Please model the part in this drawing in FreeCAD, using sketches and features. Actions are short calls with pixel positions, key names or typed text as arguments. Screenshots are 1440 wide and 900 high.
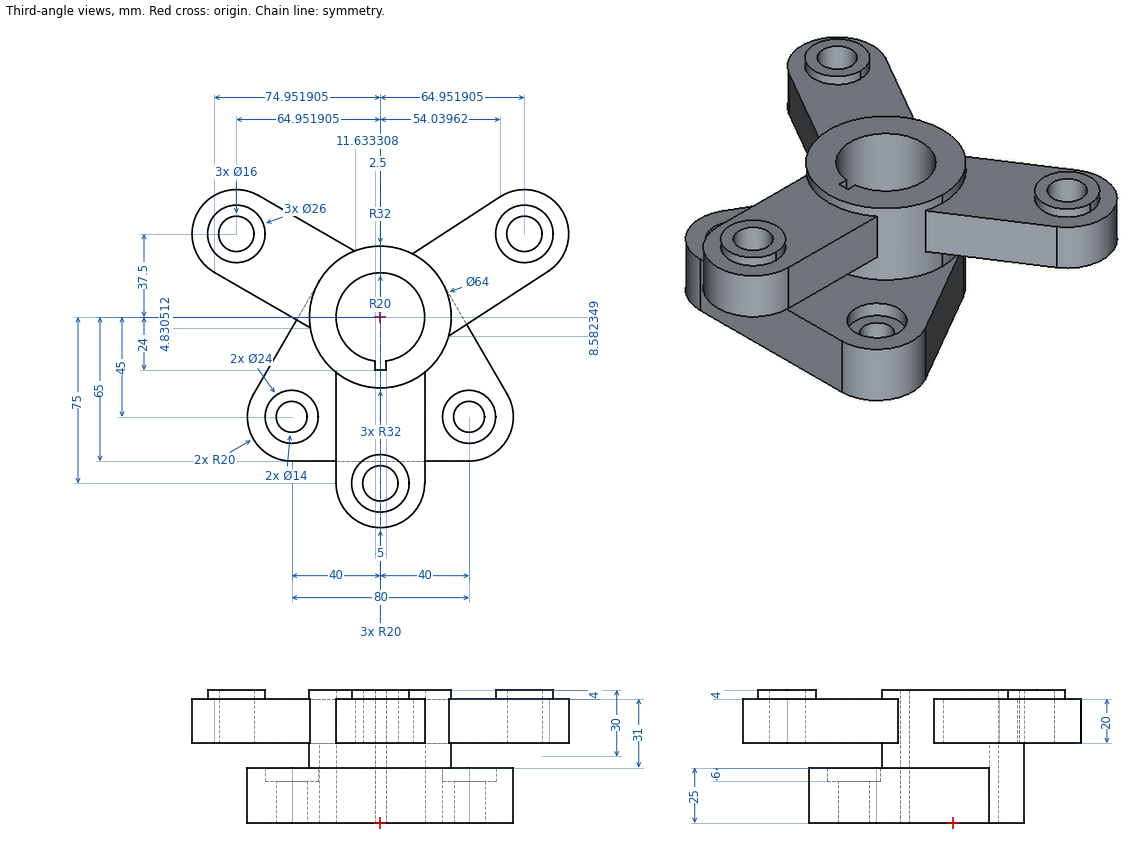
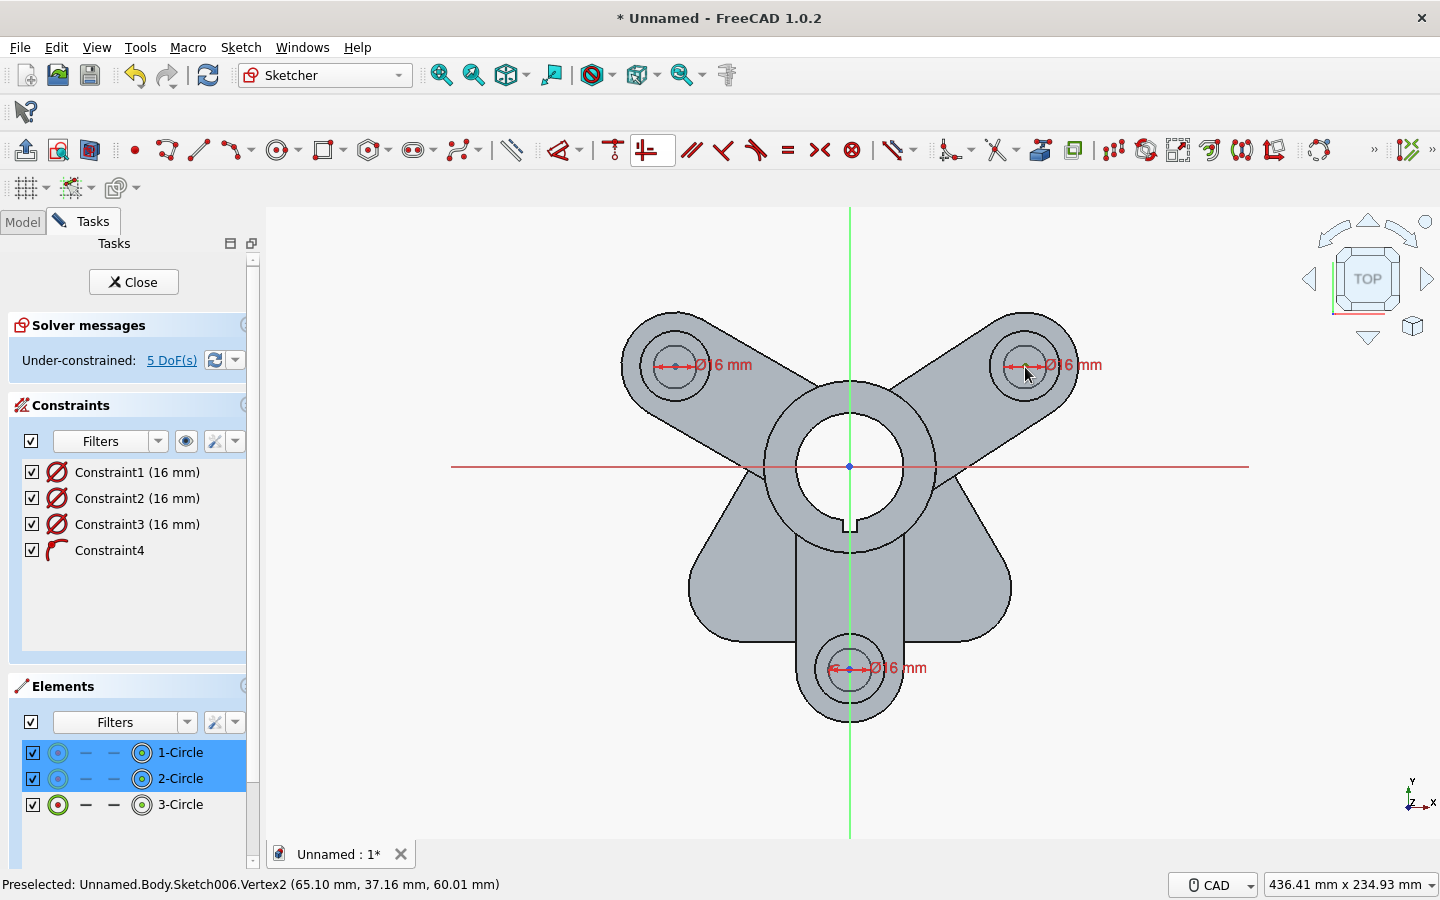
key(h)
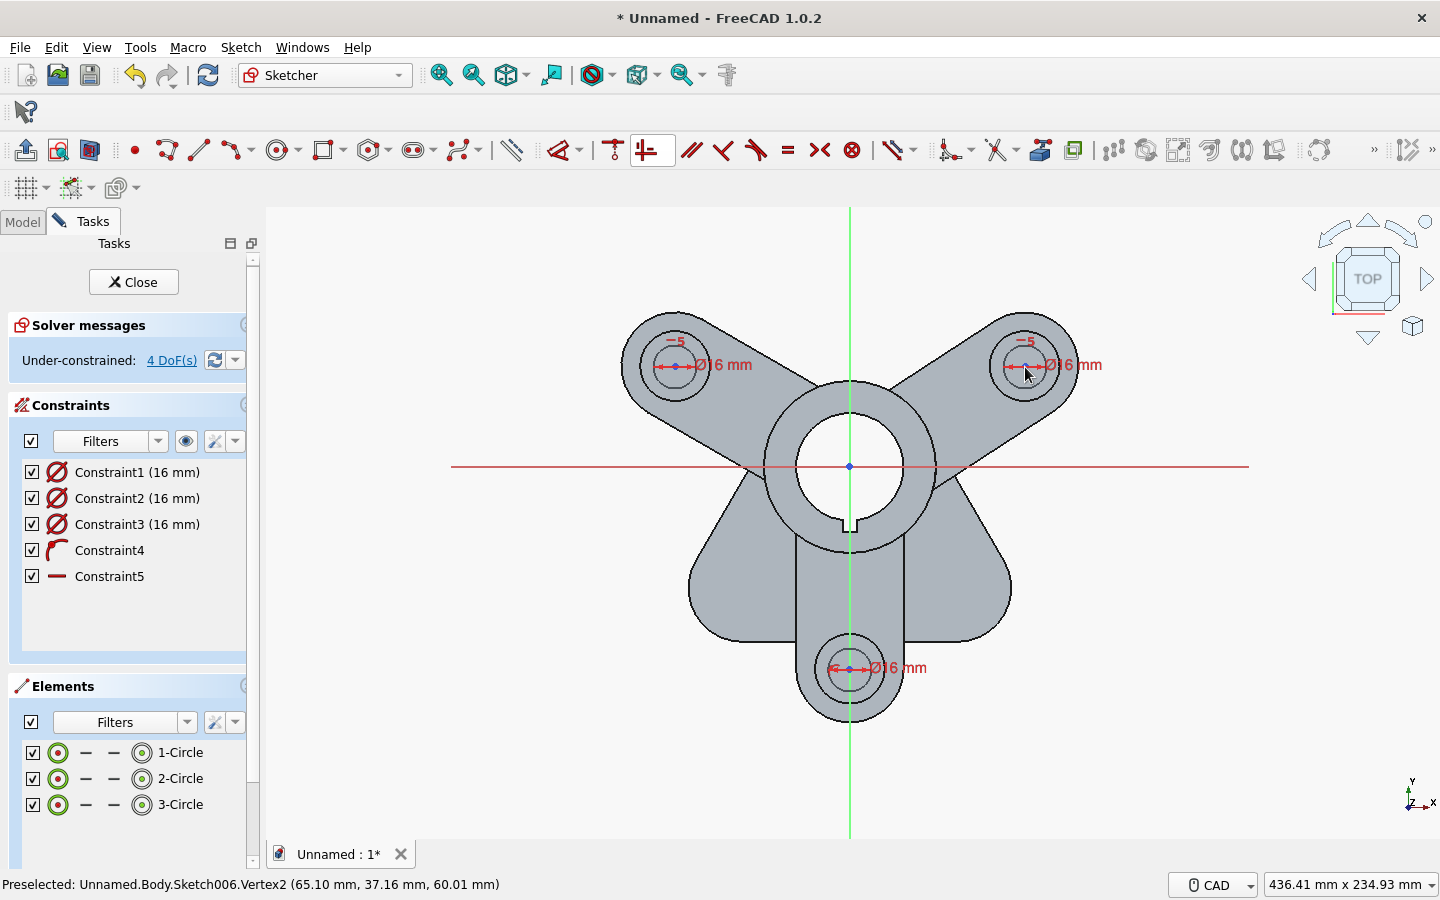
click(558, 150)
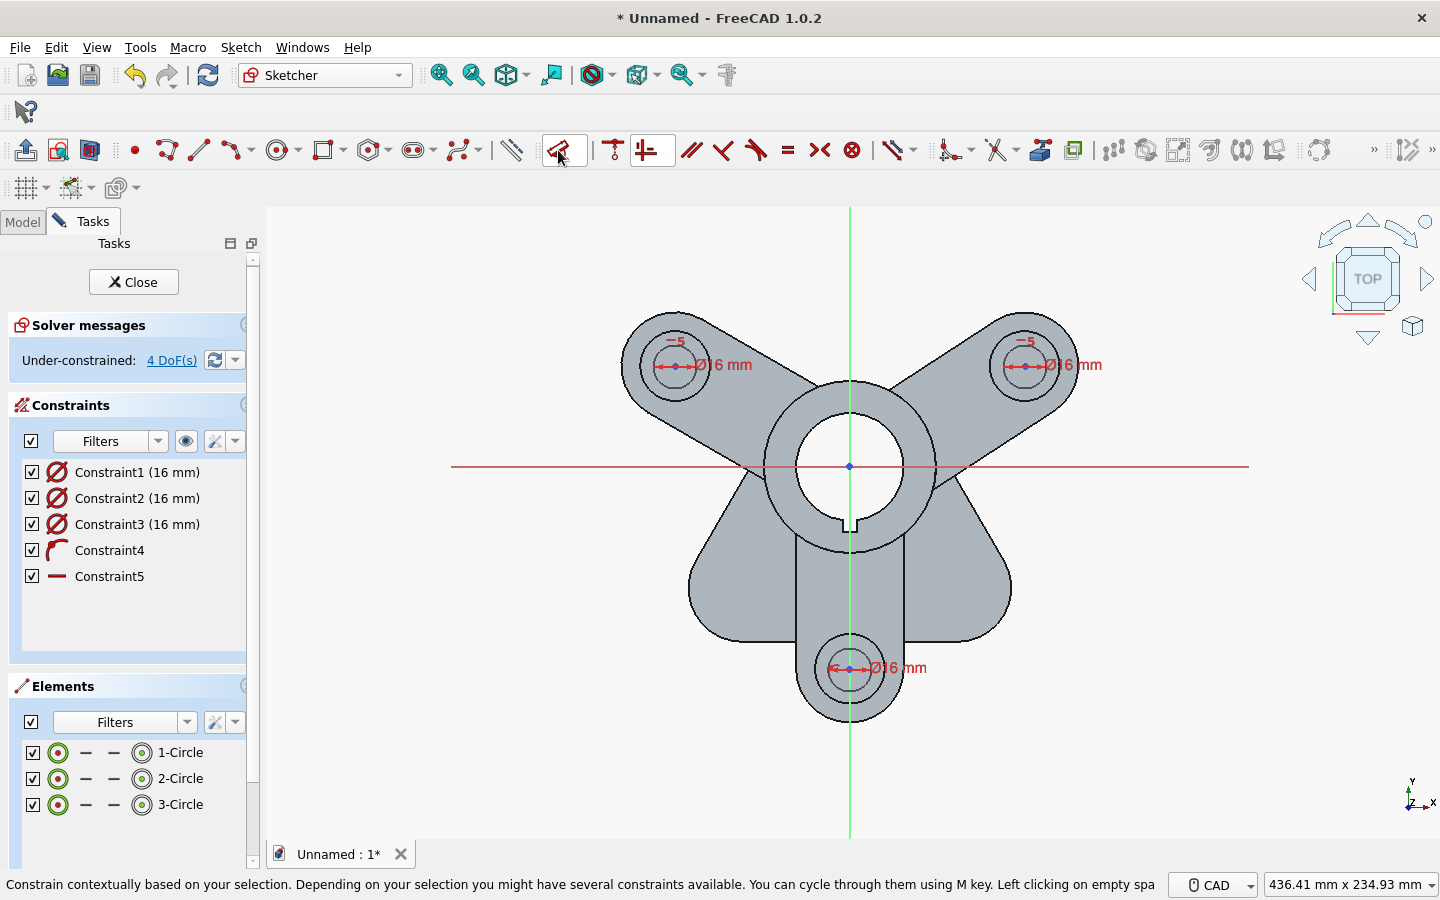
click(850, 670)
click(884, 568)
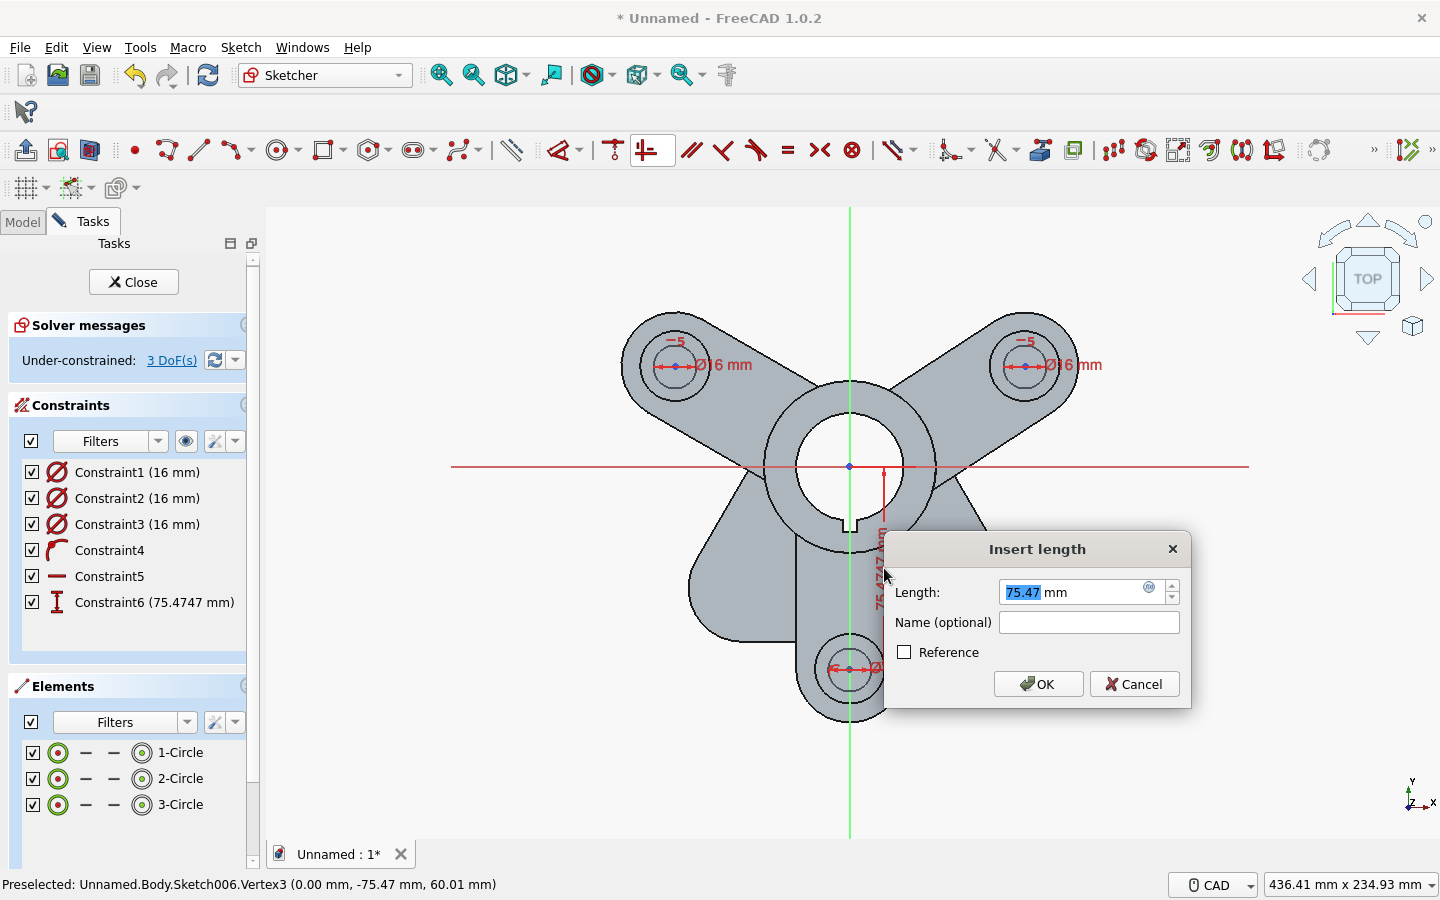
text(75)
key(Return)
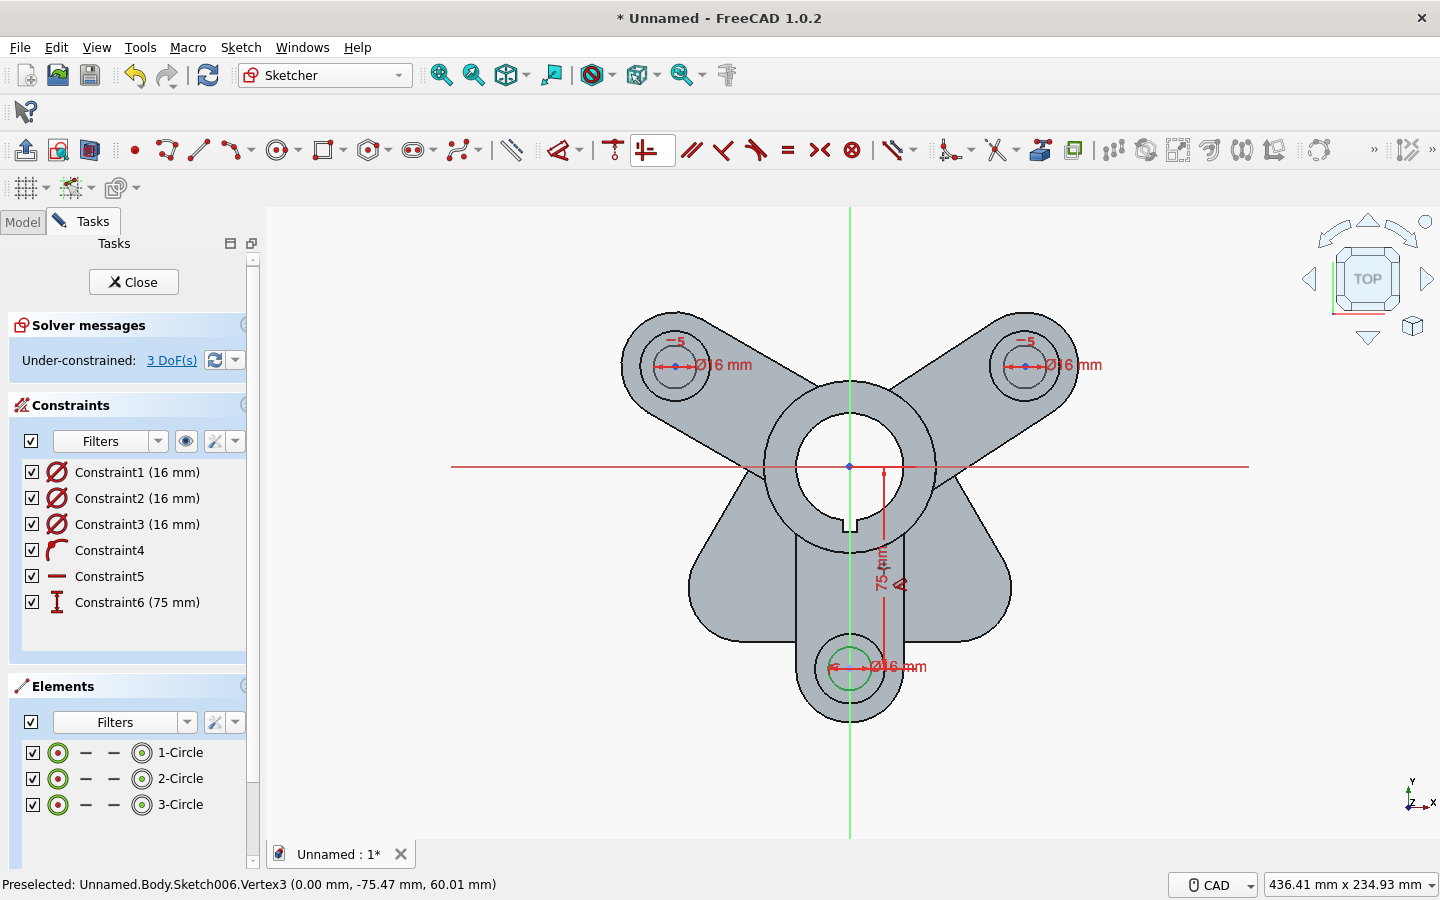
click(675, 367)
click(641, 417)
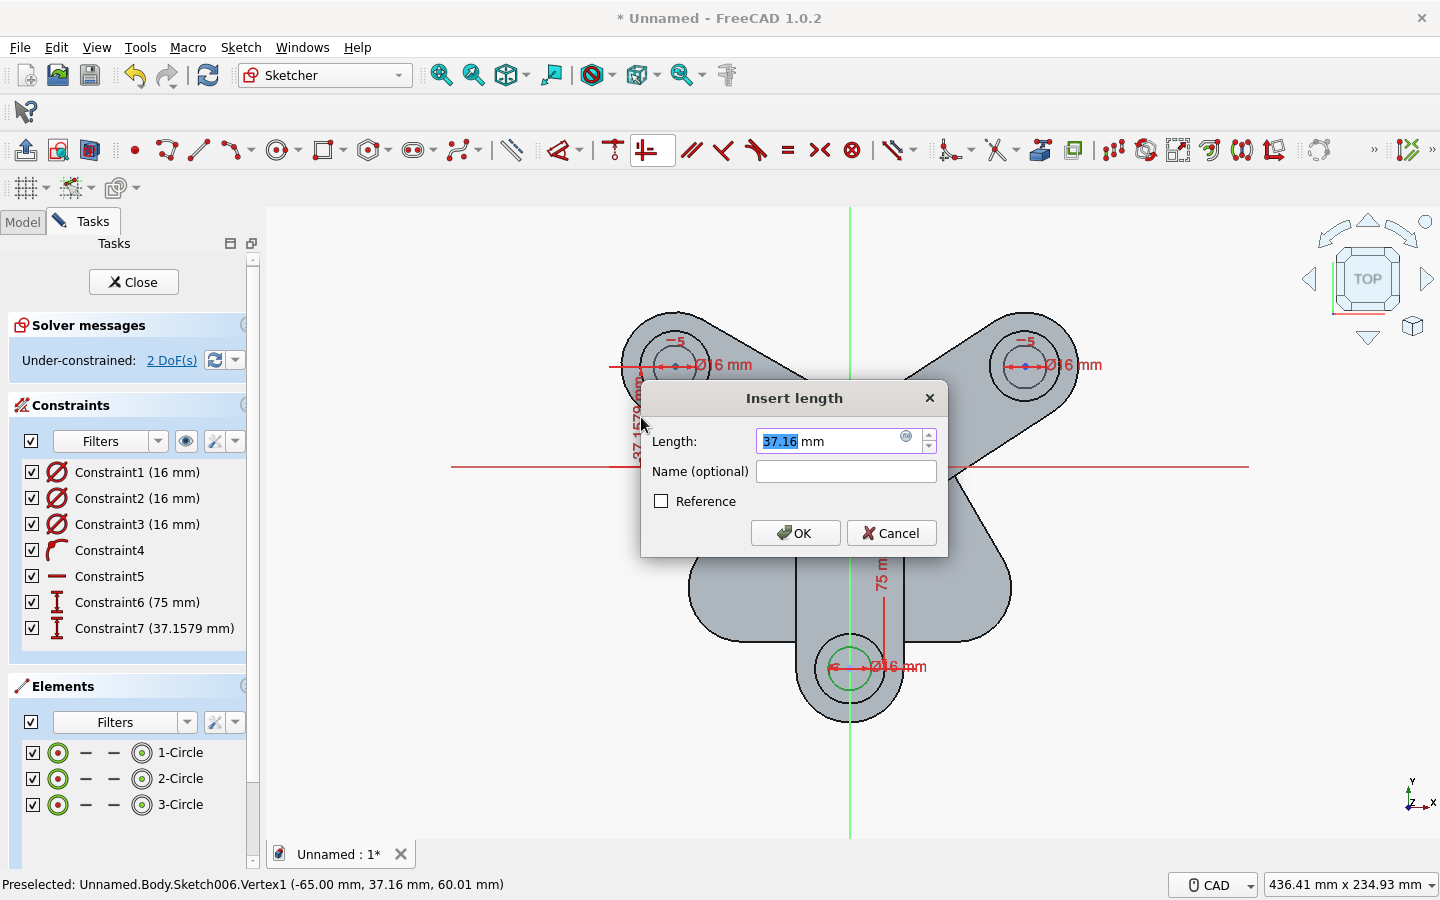
text(37.5)
key(Return)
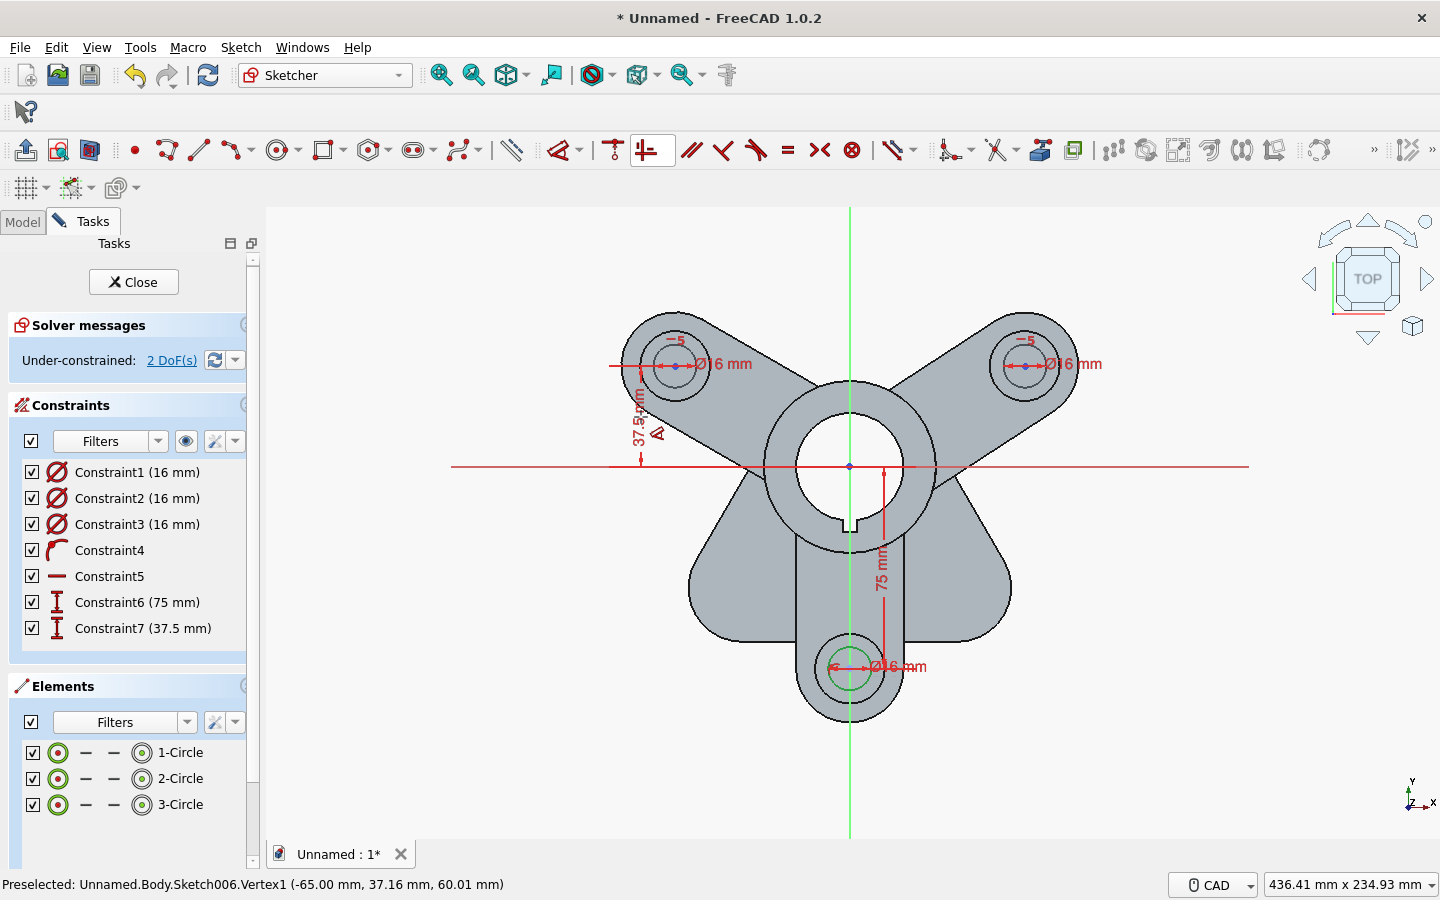
click(675, 366)
click(762, 332)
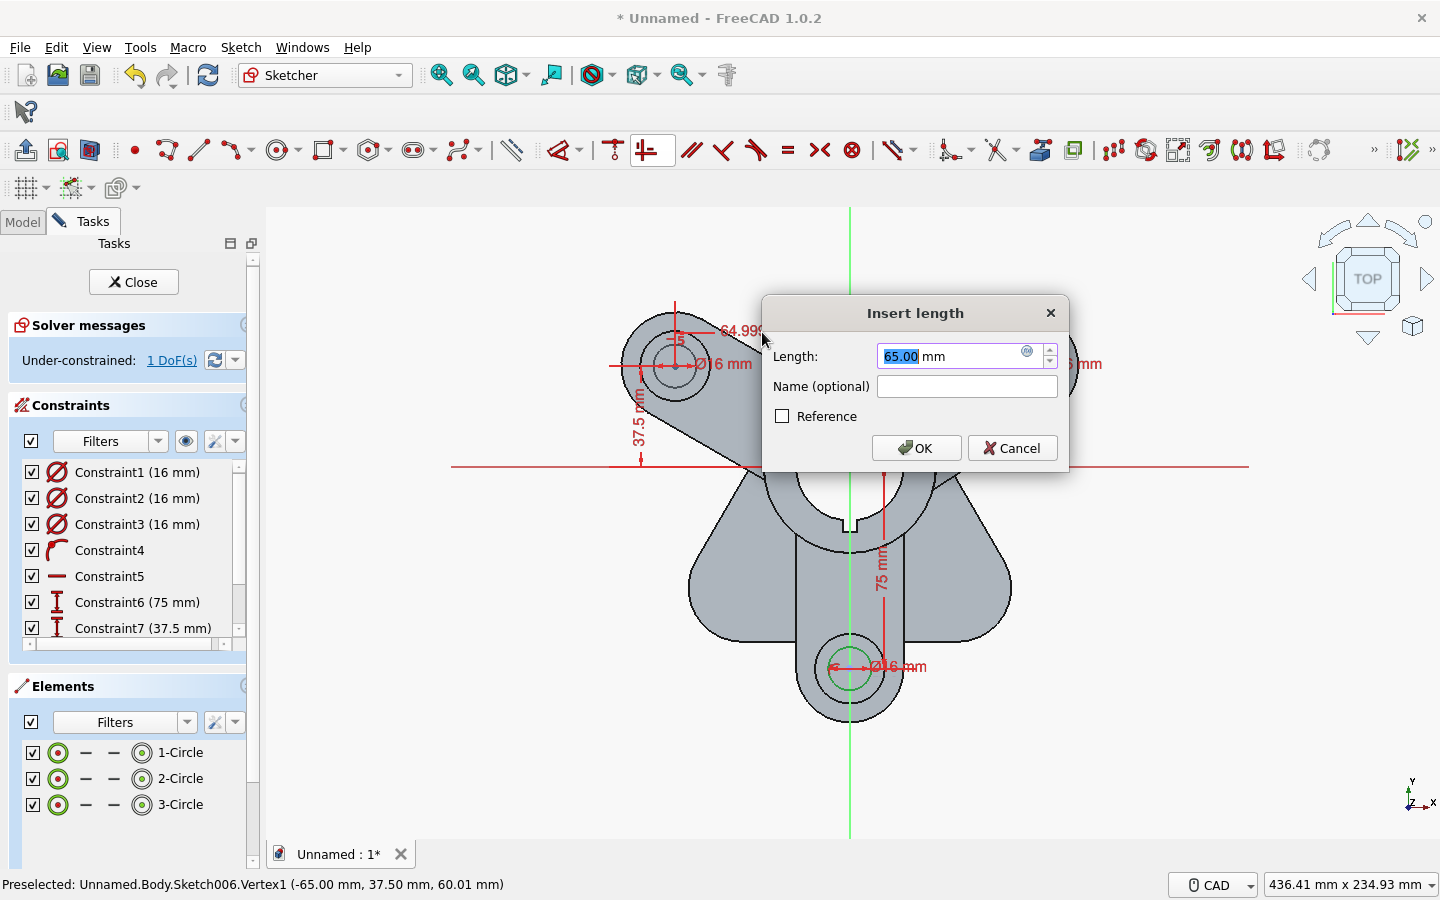
text(64.951905)
key(Return)